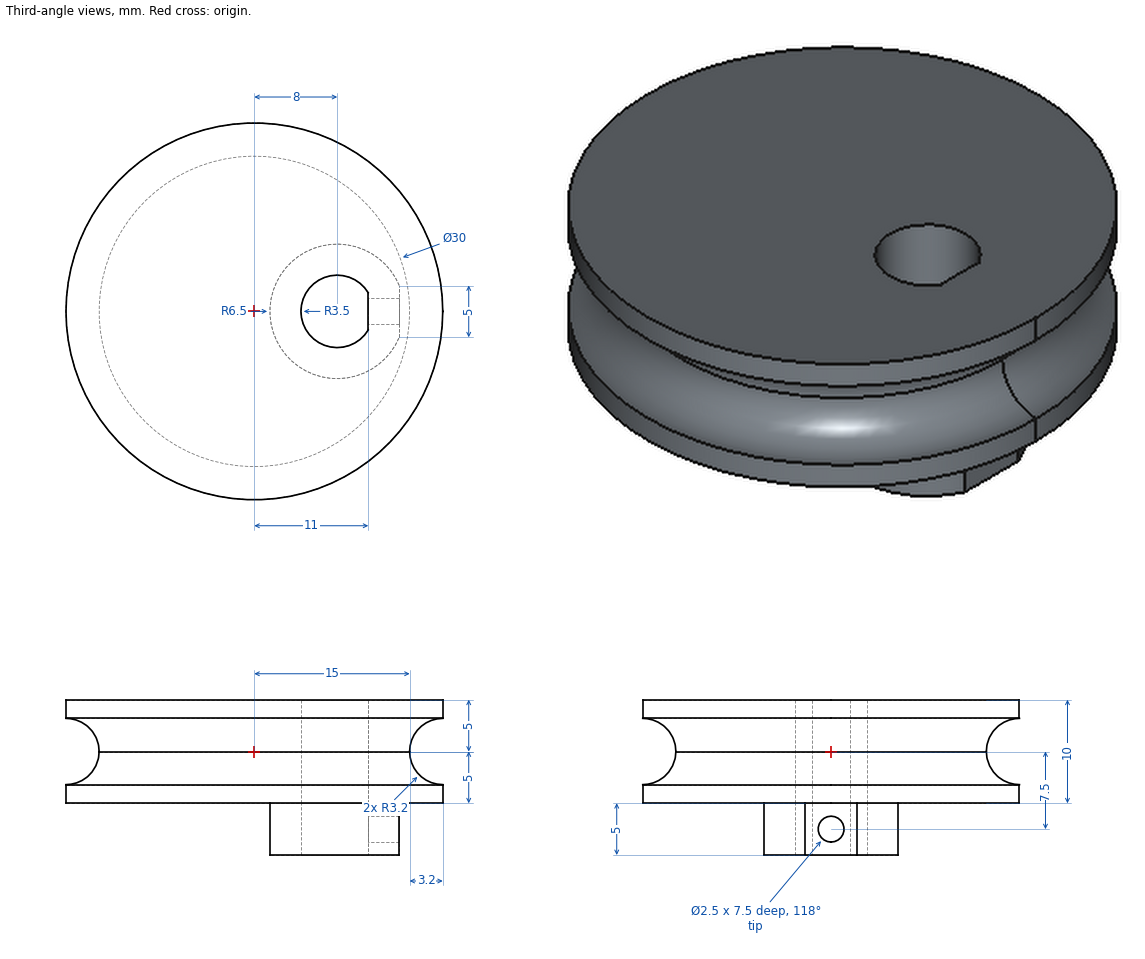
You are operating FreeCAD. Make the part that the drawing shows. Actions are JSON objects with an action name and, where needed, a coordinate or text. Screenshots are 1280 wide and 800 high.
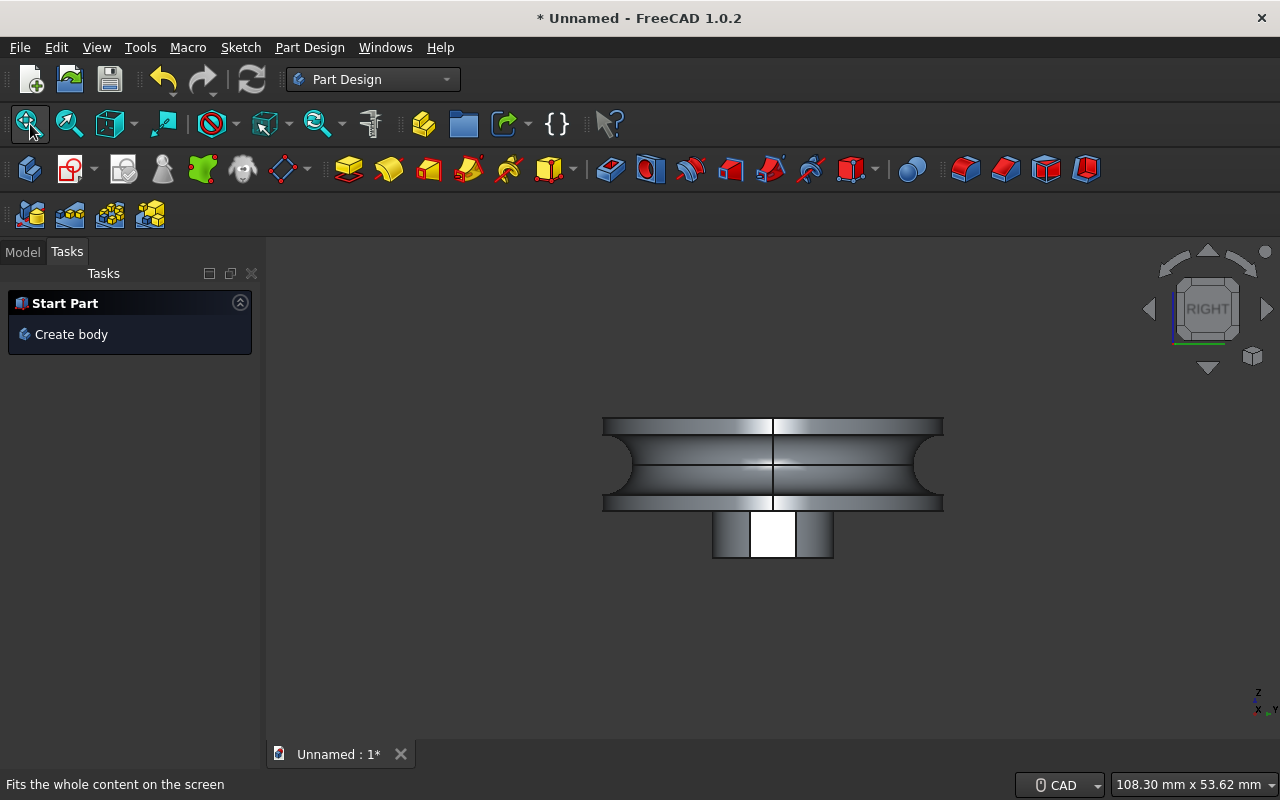
{"action": "left_click", "coordinate": [773, 534]}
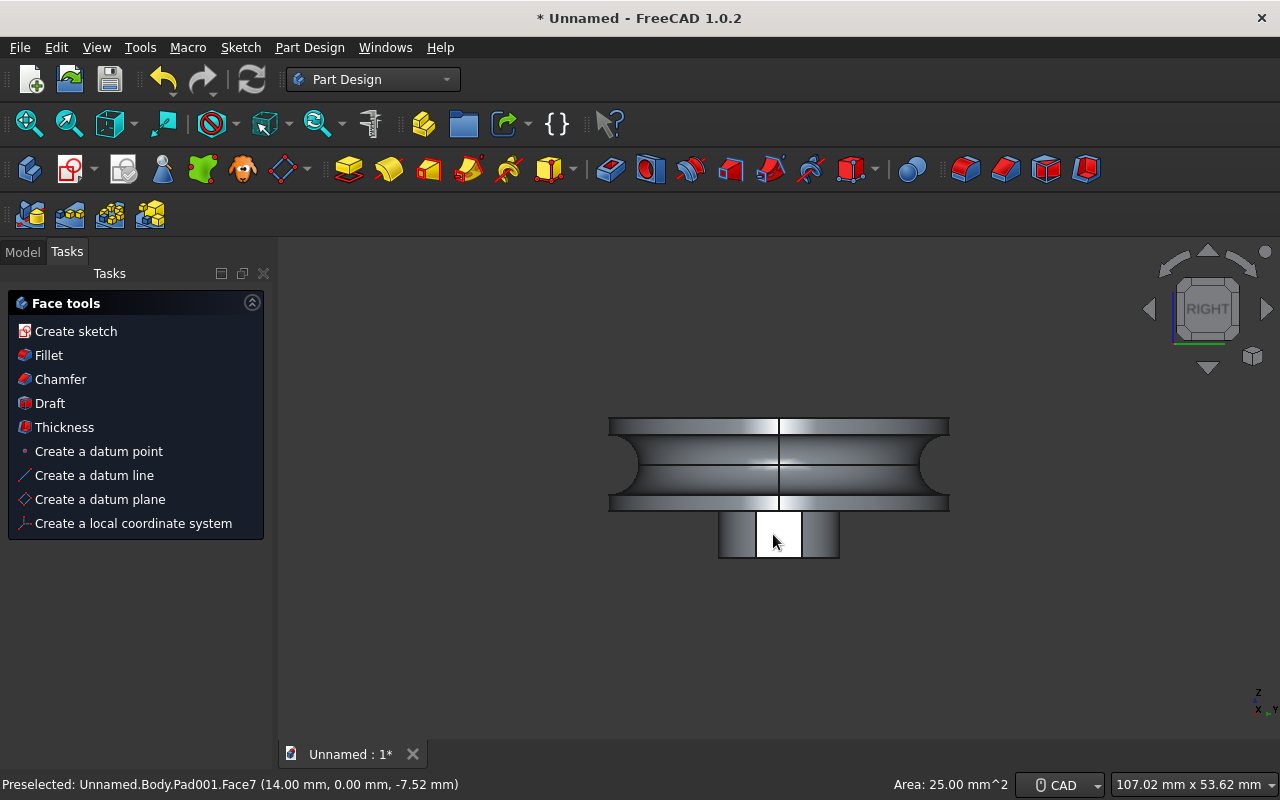
{"action": "left_click", "coordinate": [70, 170]}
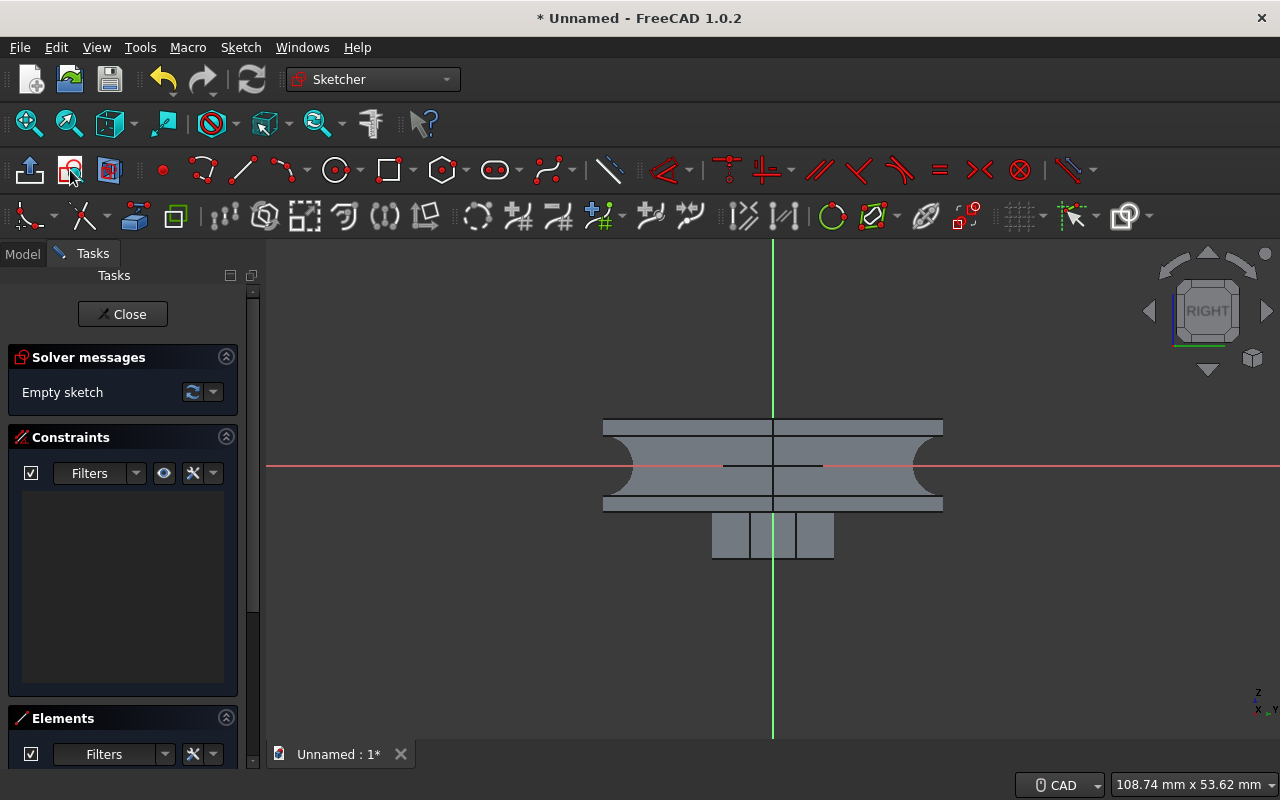
{"action": "left_click", "coordinate": [110, 170]}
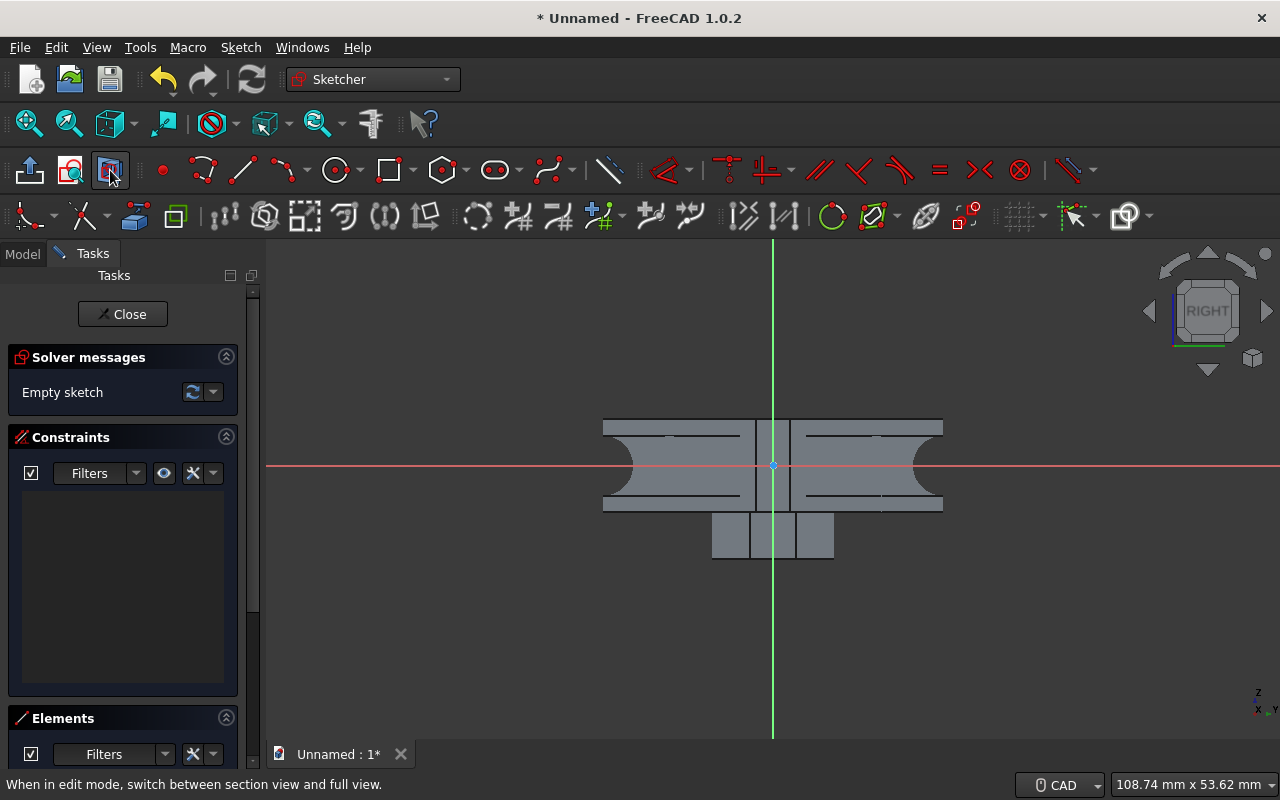
{"action": "scroll", "coordinate": [778, 539], "scroll_direction": "up", "scroll_amount": 13}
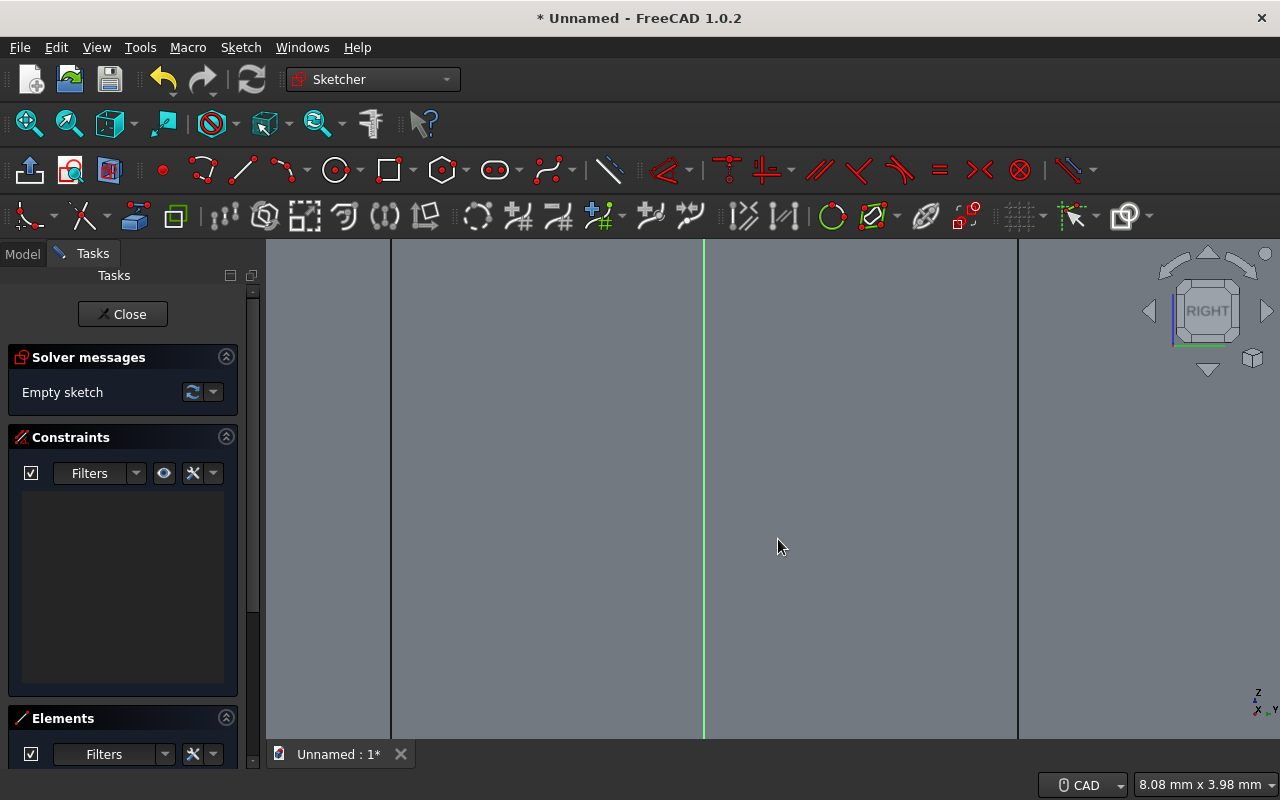
{"action": "left_click", "coordinate": [336, 170]}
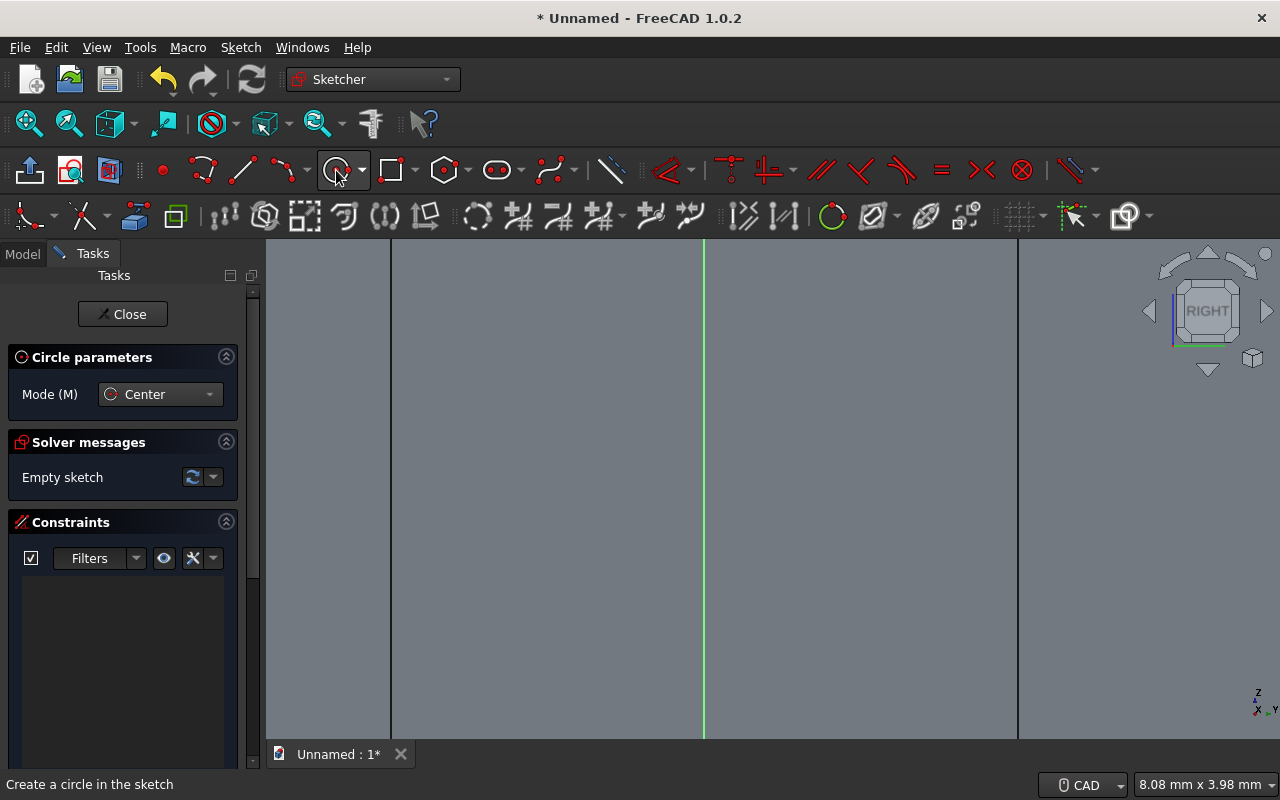
{"action": "left_click", "coordinate": [704, 486]}
{"action": "mouse_move", "coordinate": [815, 375]}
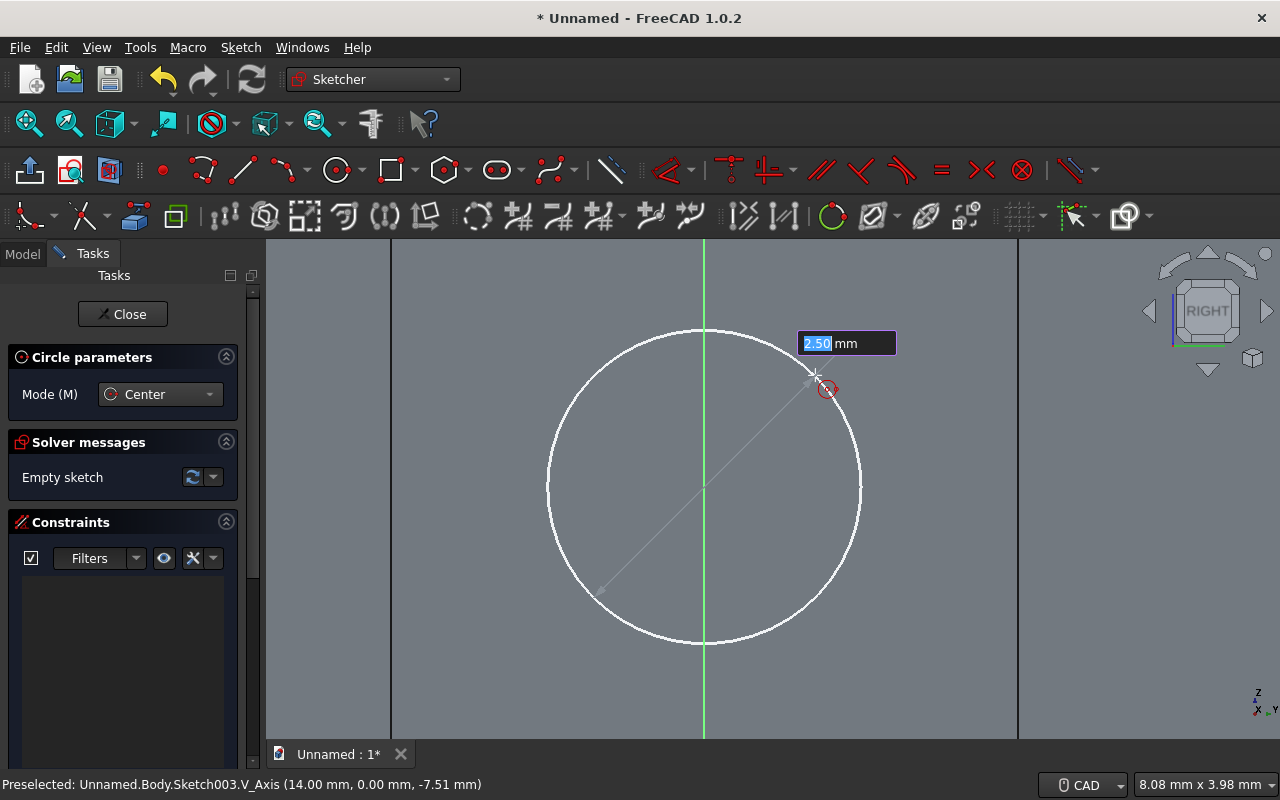
{"action": "type", "text": "2.5"}
{"action": "key", "text": "Return"}
{"action": "key", "text": "Escape"}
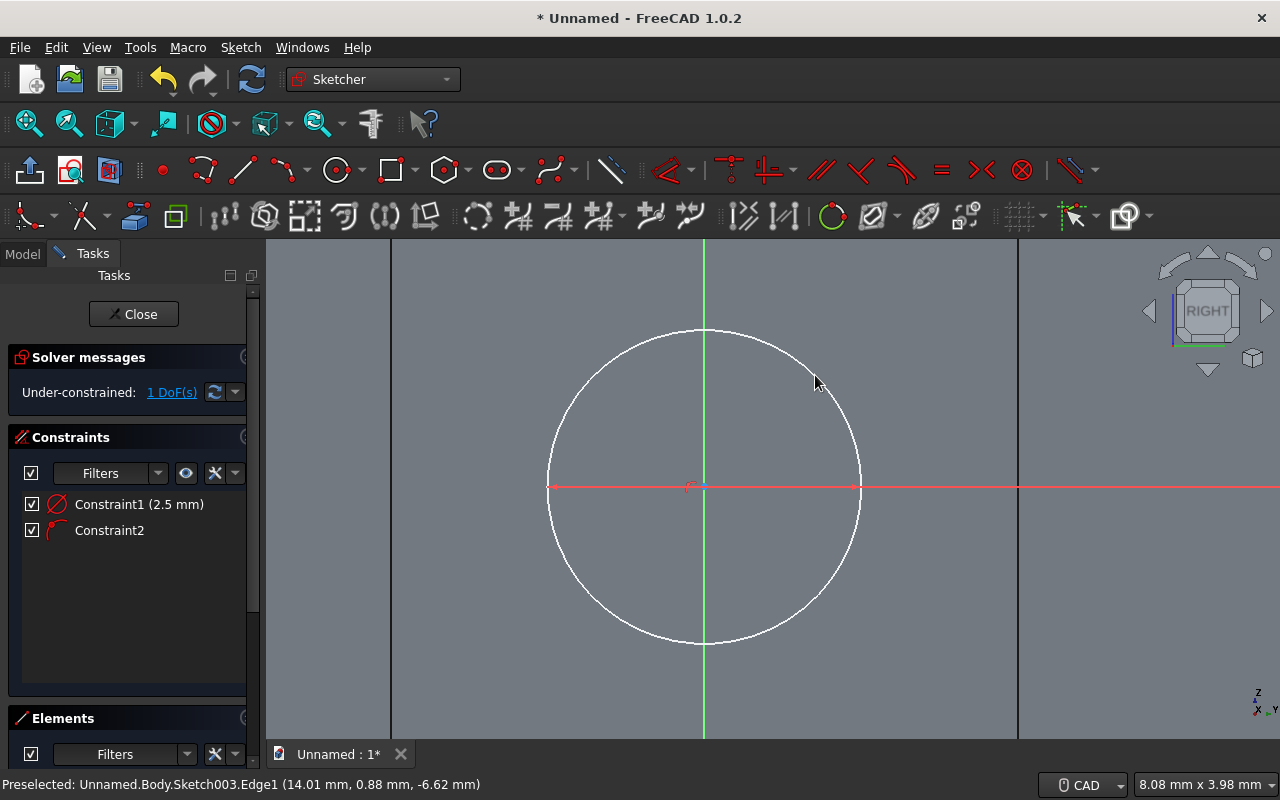
{"action": "left_click", "coordinate": [666, 170]}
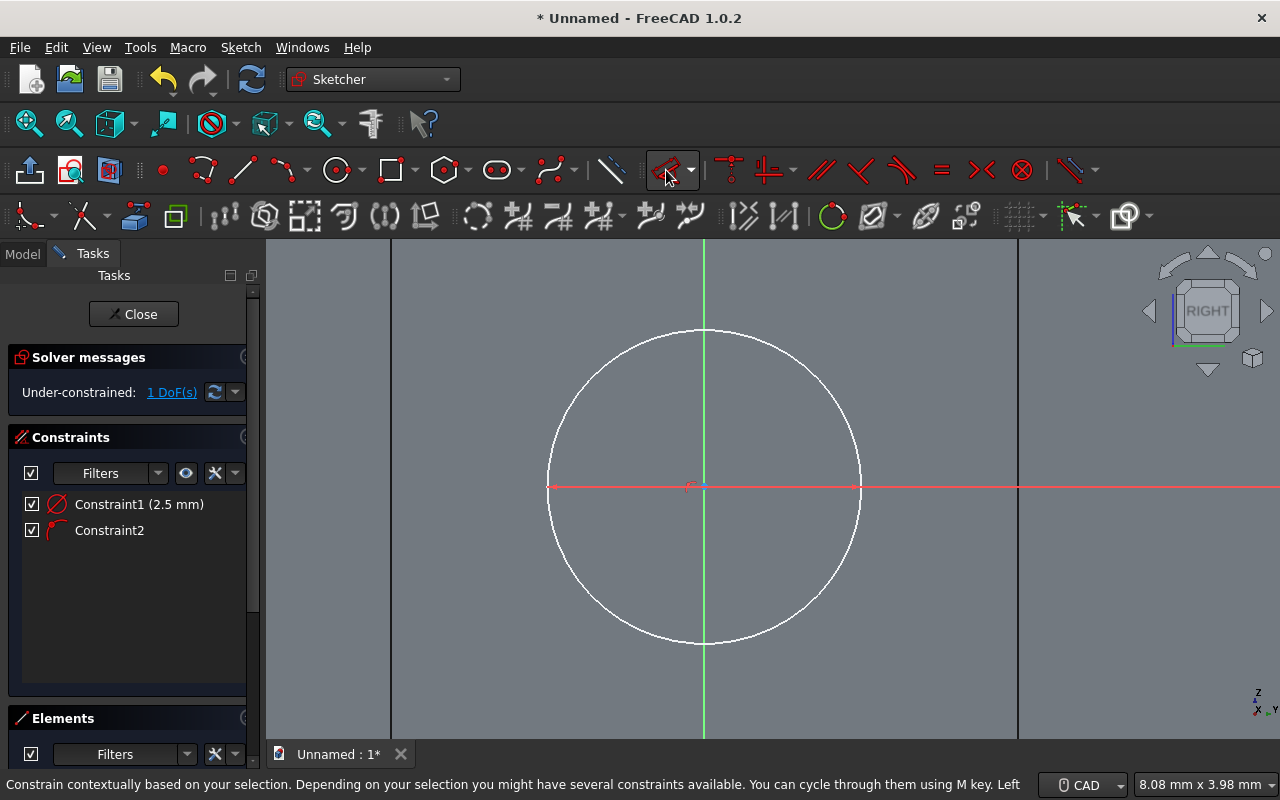
{"action": "left_click", "coordinate": [704, 487]}
{"action": "left_click", "coordinate": [738, 377]}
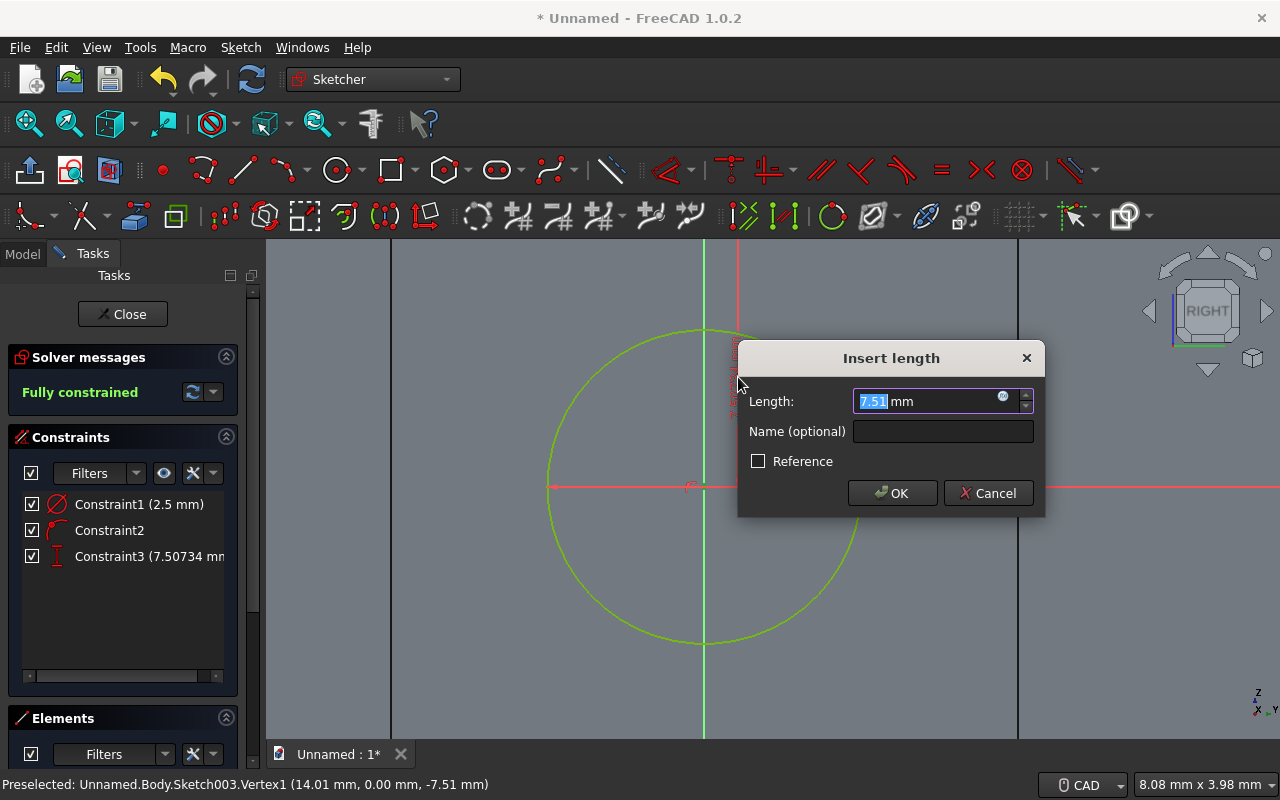
{"action": "type", "text": "7.5"}
{"action": "key", "text": "Return"}
{"action": "key", "text": "Escape"}